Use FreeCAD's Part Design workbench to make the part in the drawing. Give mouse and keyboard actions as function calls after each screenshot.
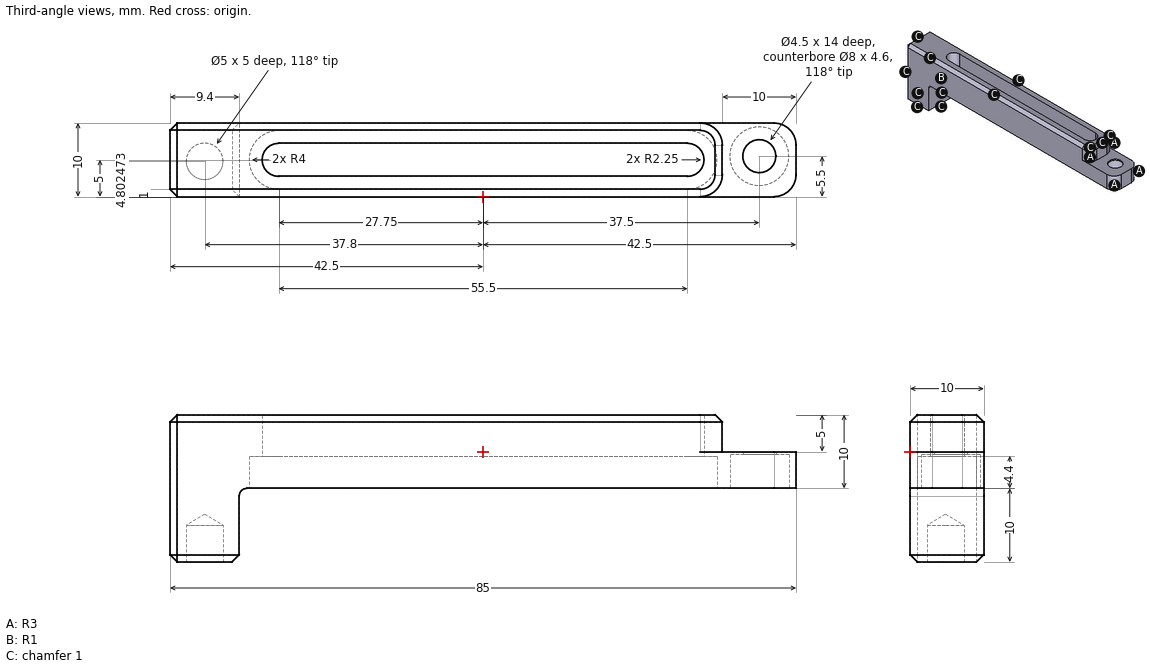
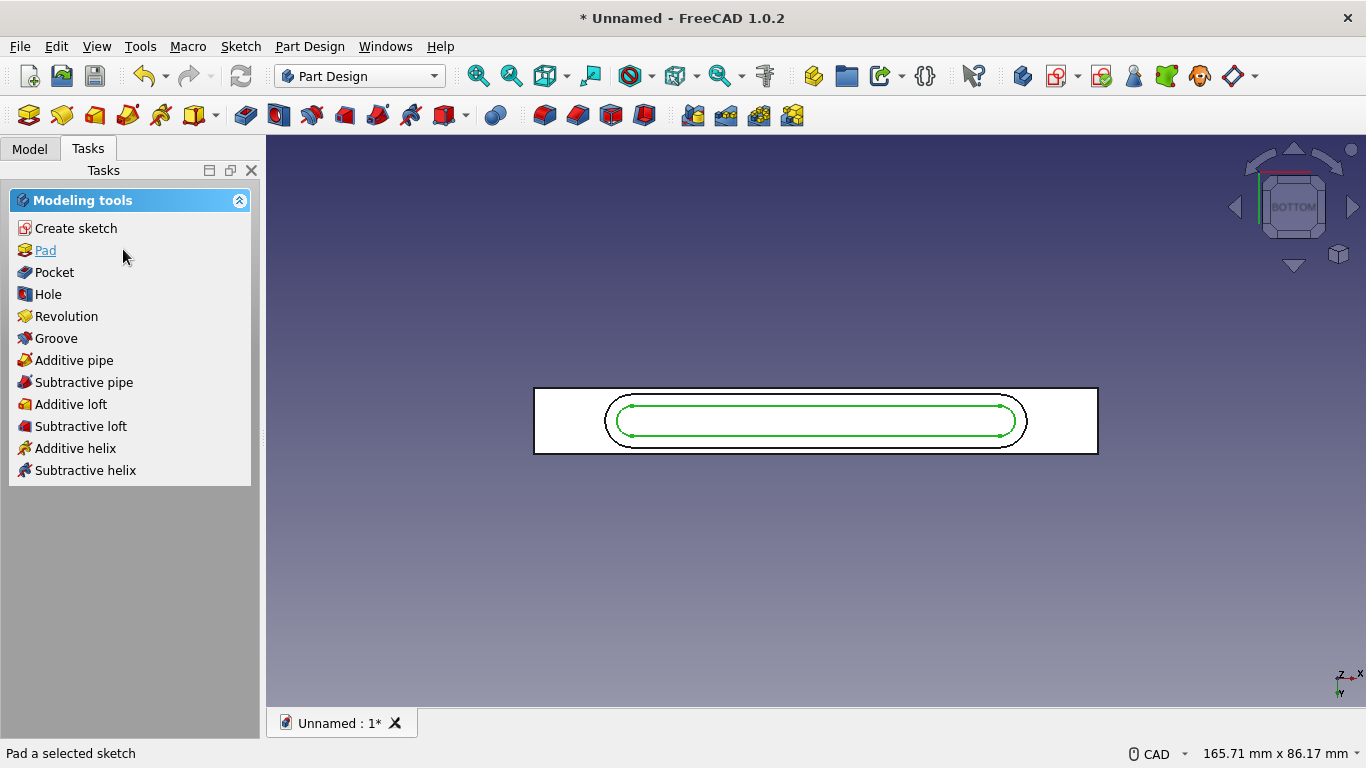
click(246, 116)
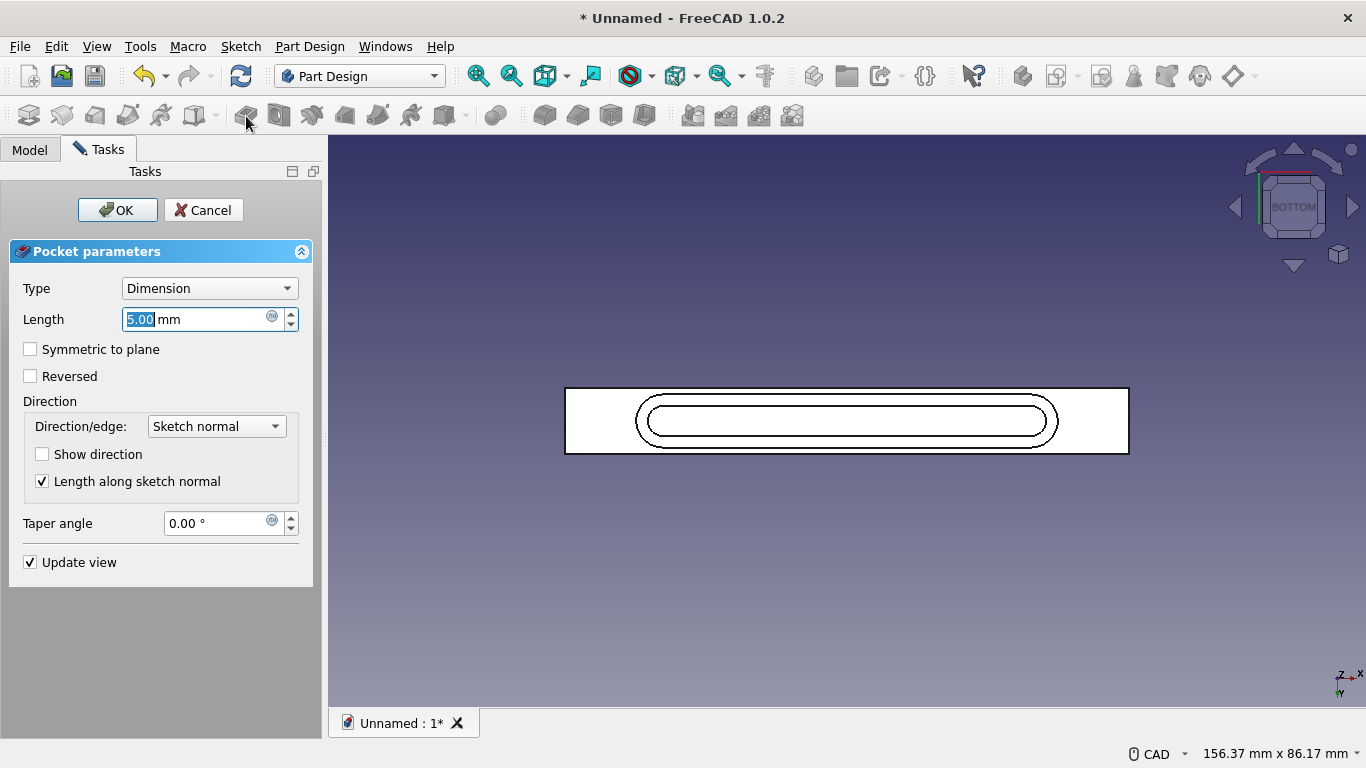
click(210, 288)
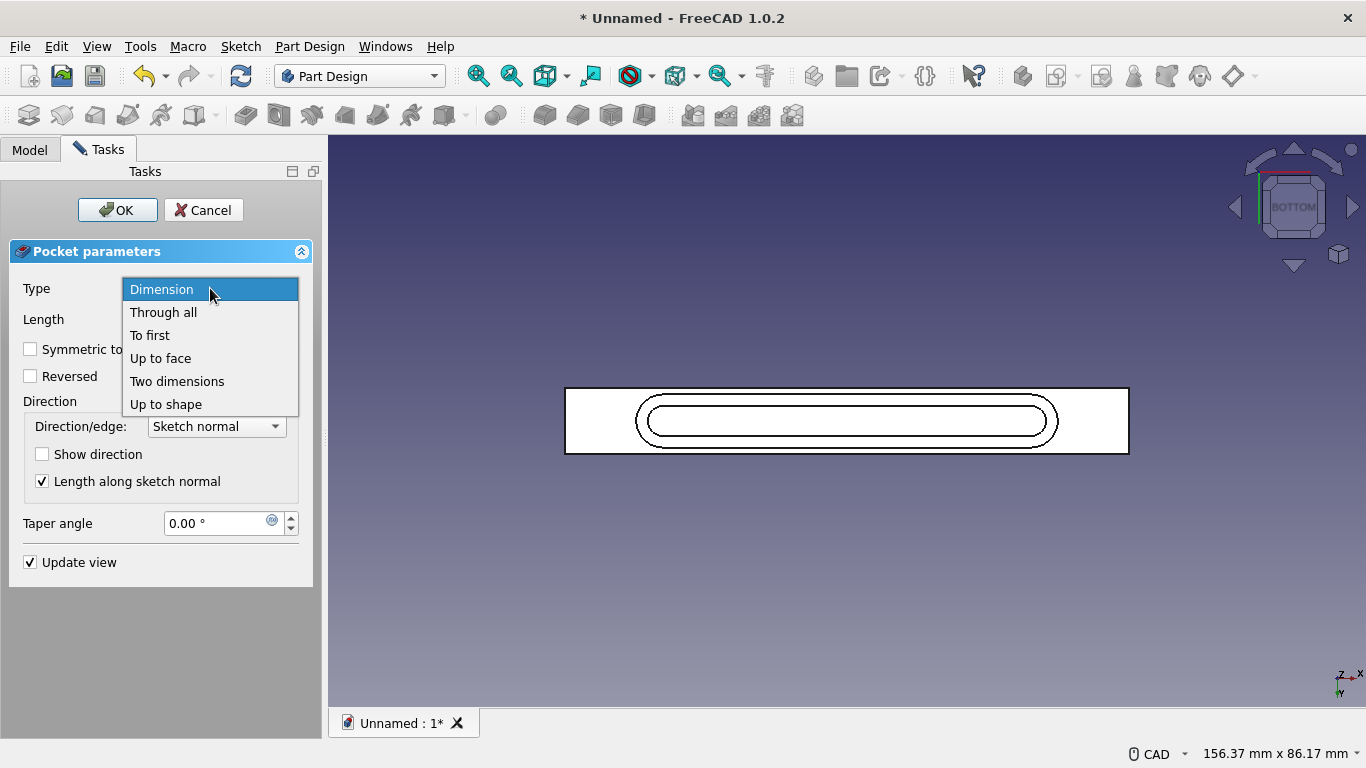
click(208, 312)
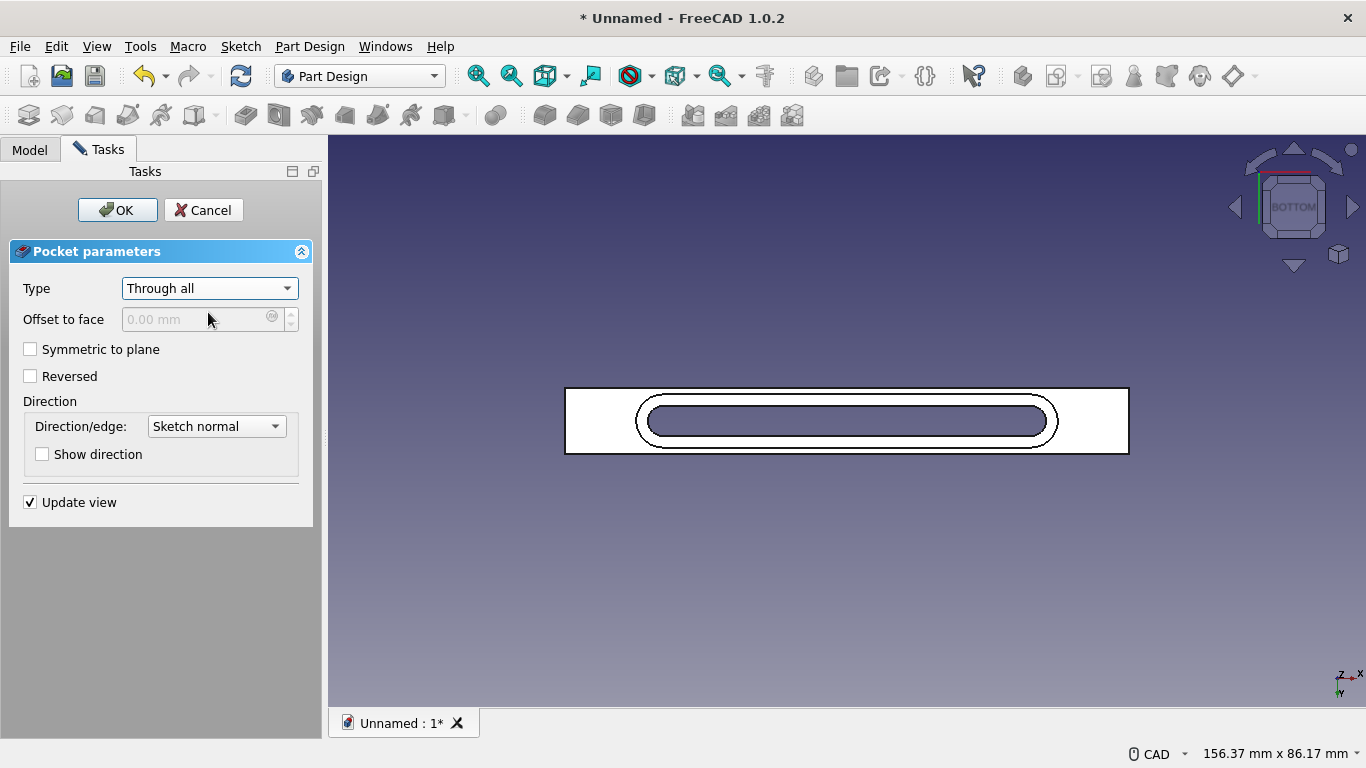
click(118, 210)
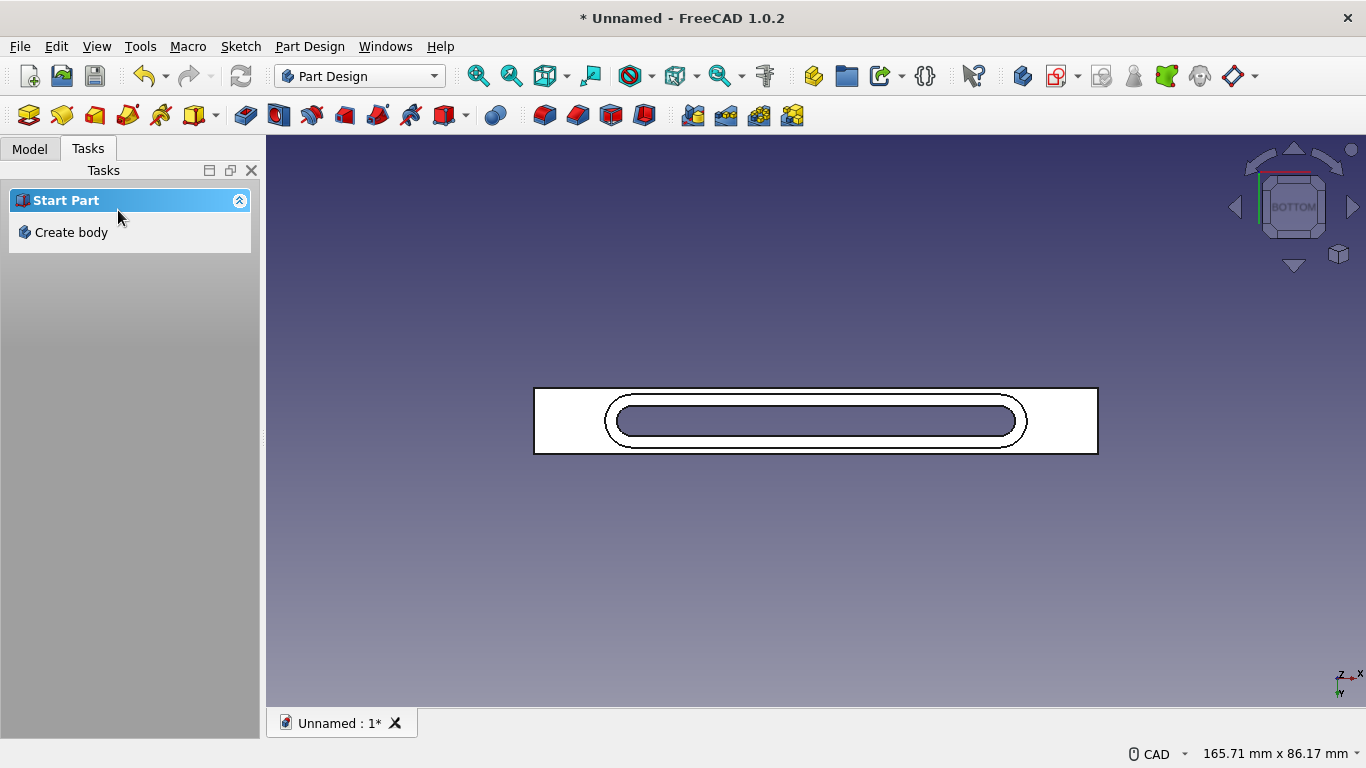
click(574, 420)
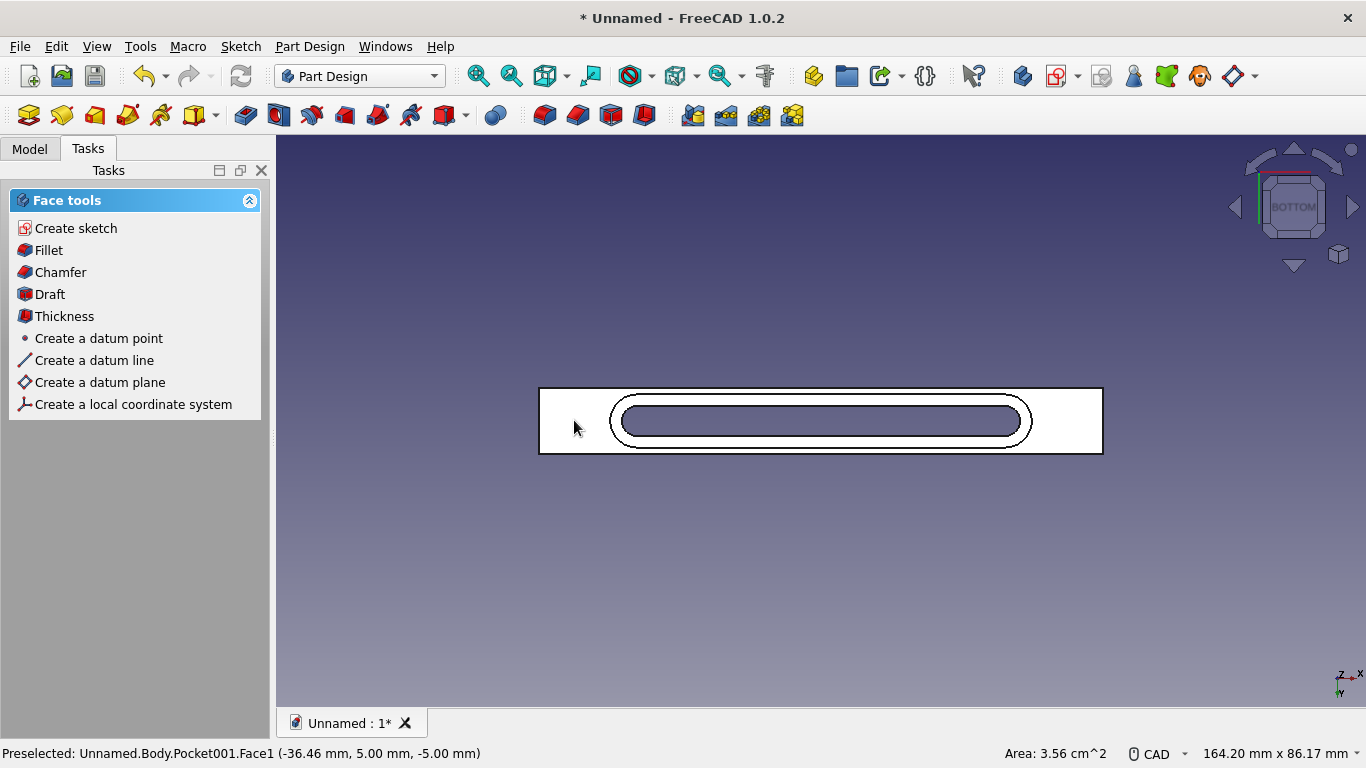
click(1056, 76)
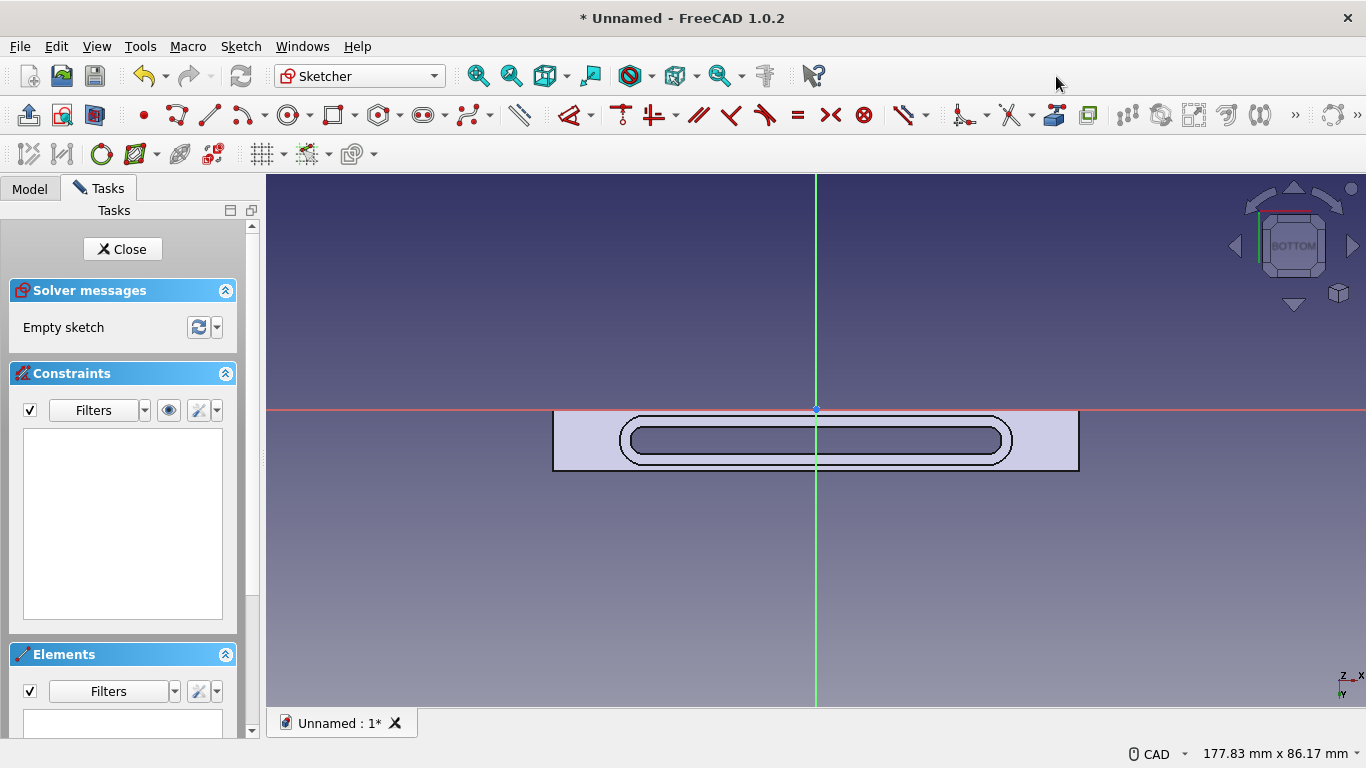
scroll(540, 441, up, 8)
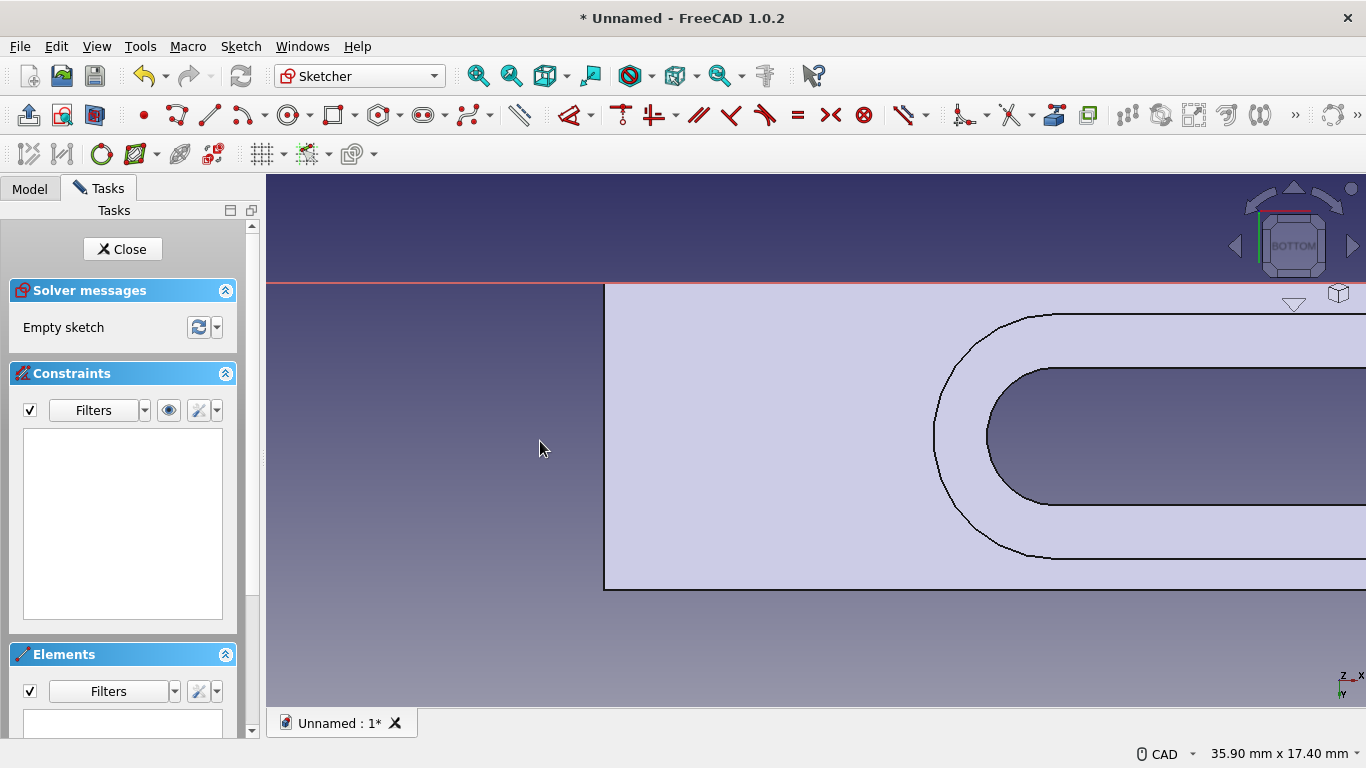
key(g)
key(r)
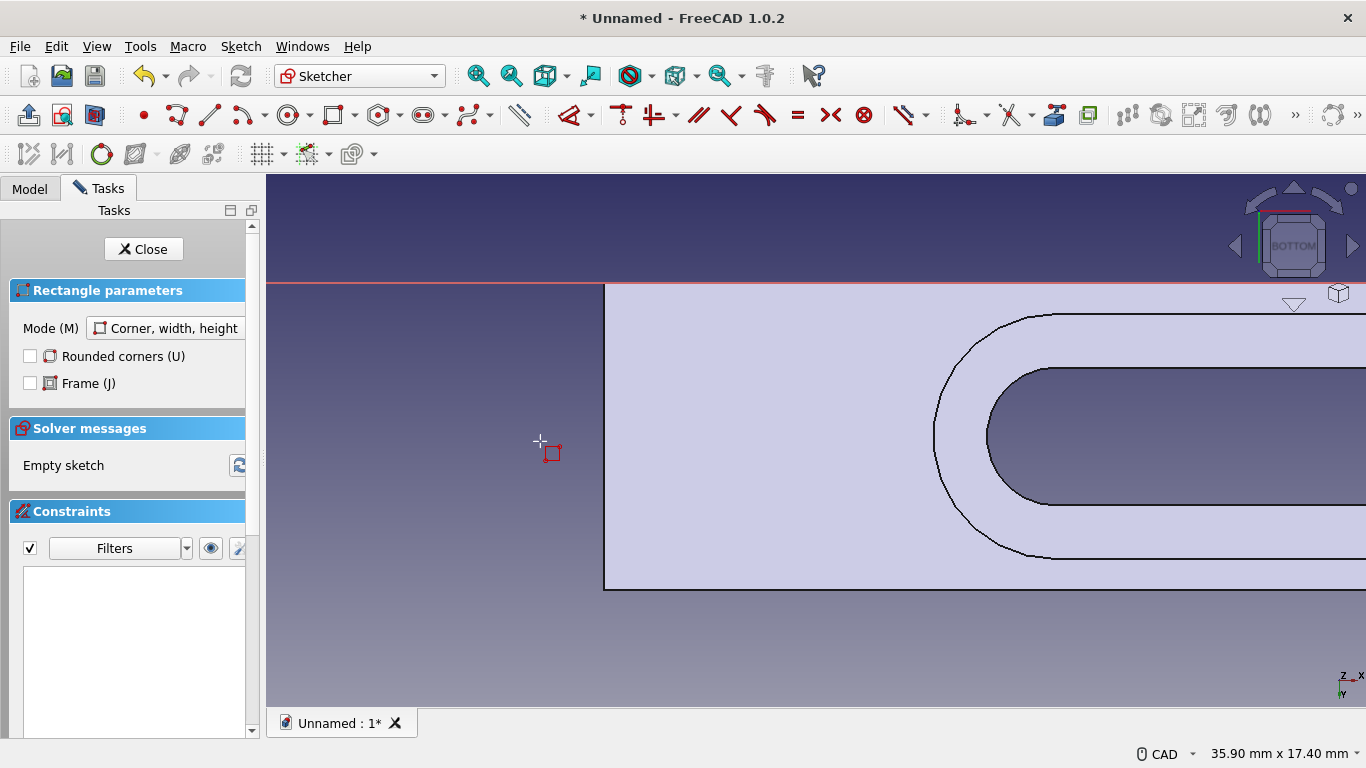
click(604, 283)
click(892, 590)
key(Escape)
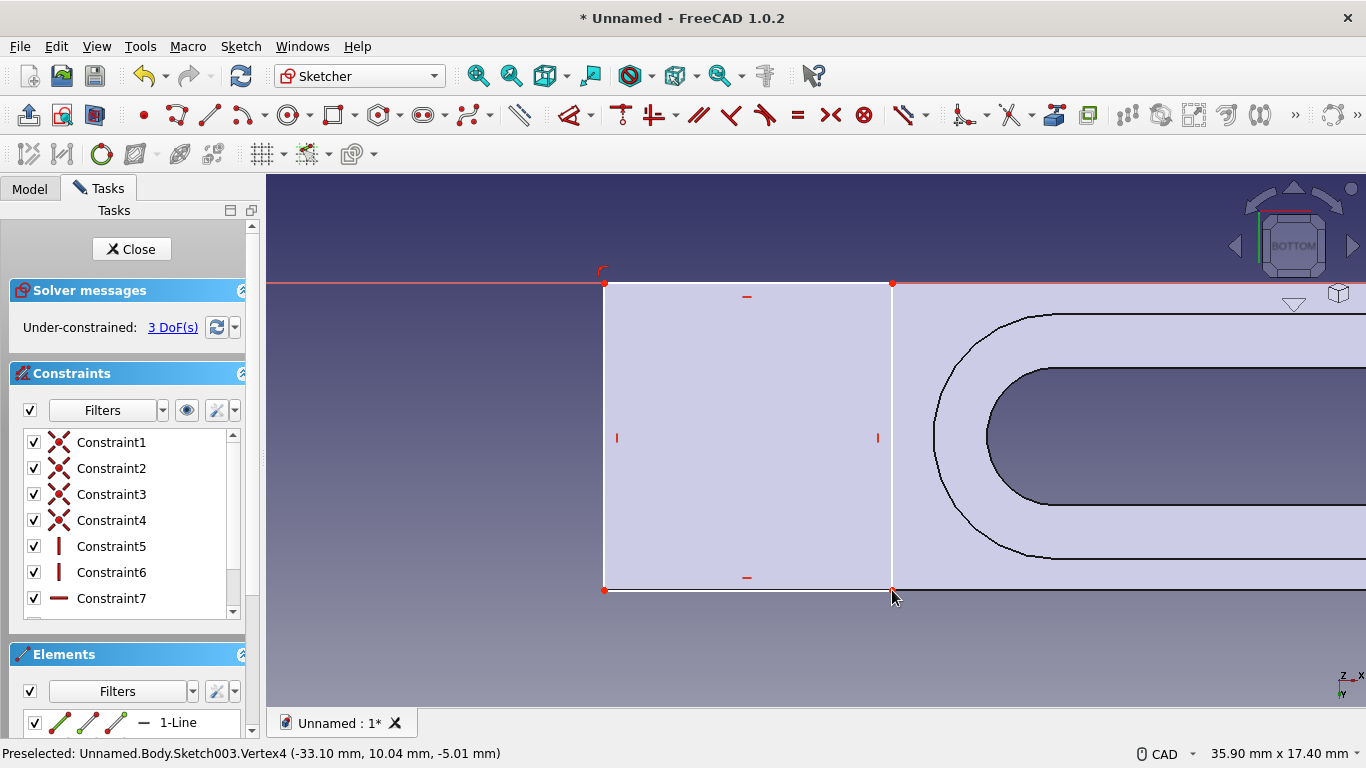
click(568, 116)